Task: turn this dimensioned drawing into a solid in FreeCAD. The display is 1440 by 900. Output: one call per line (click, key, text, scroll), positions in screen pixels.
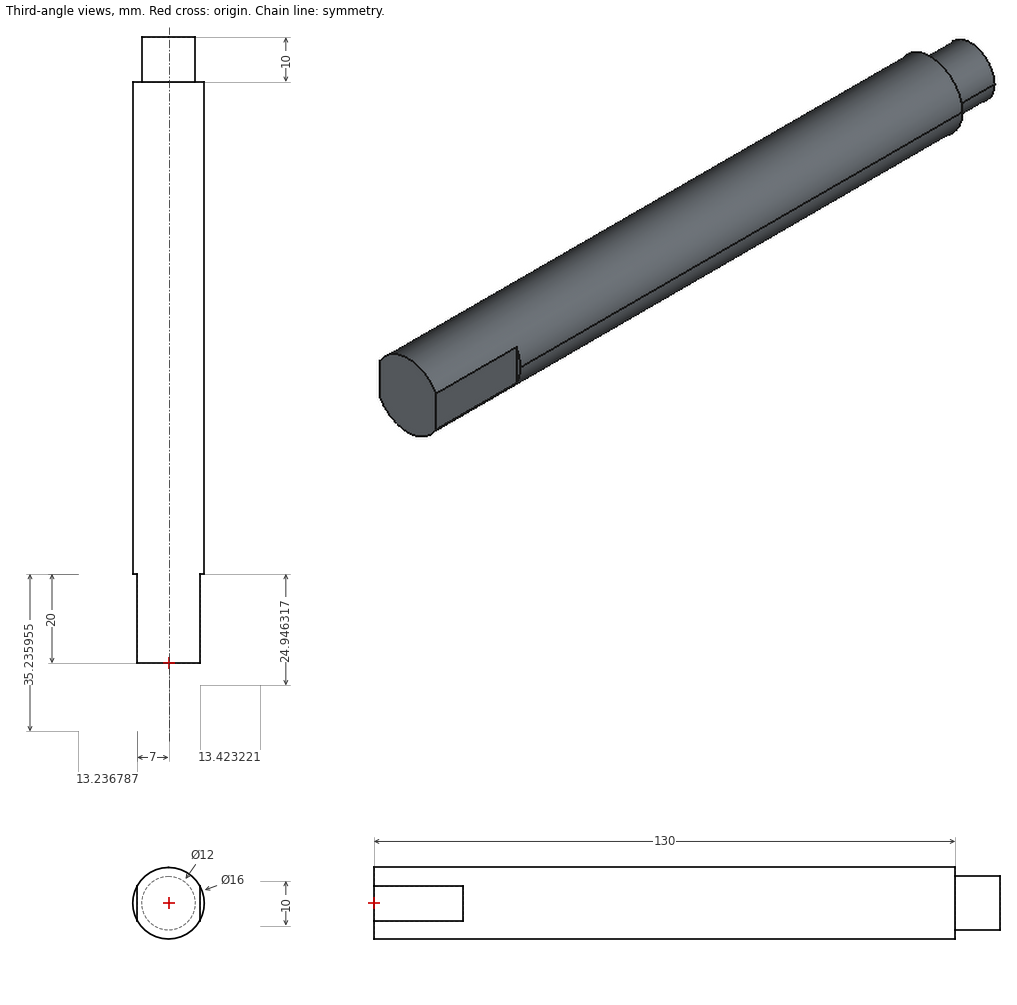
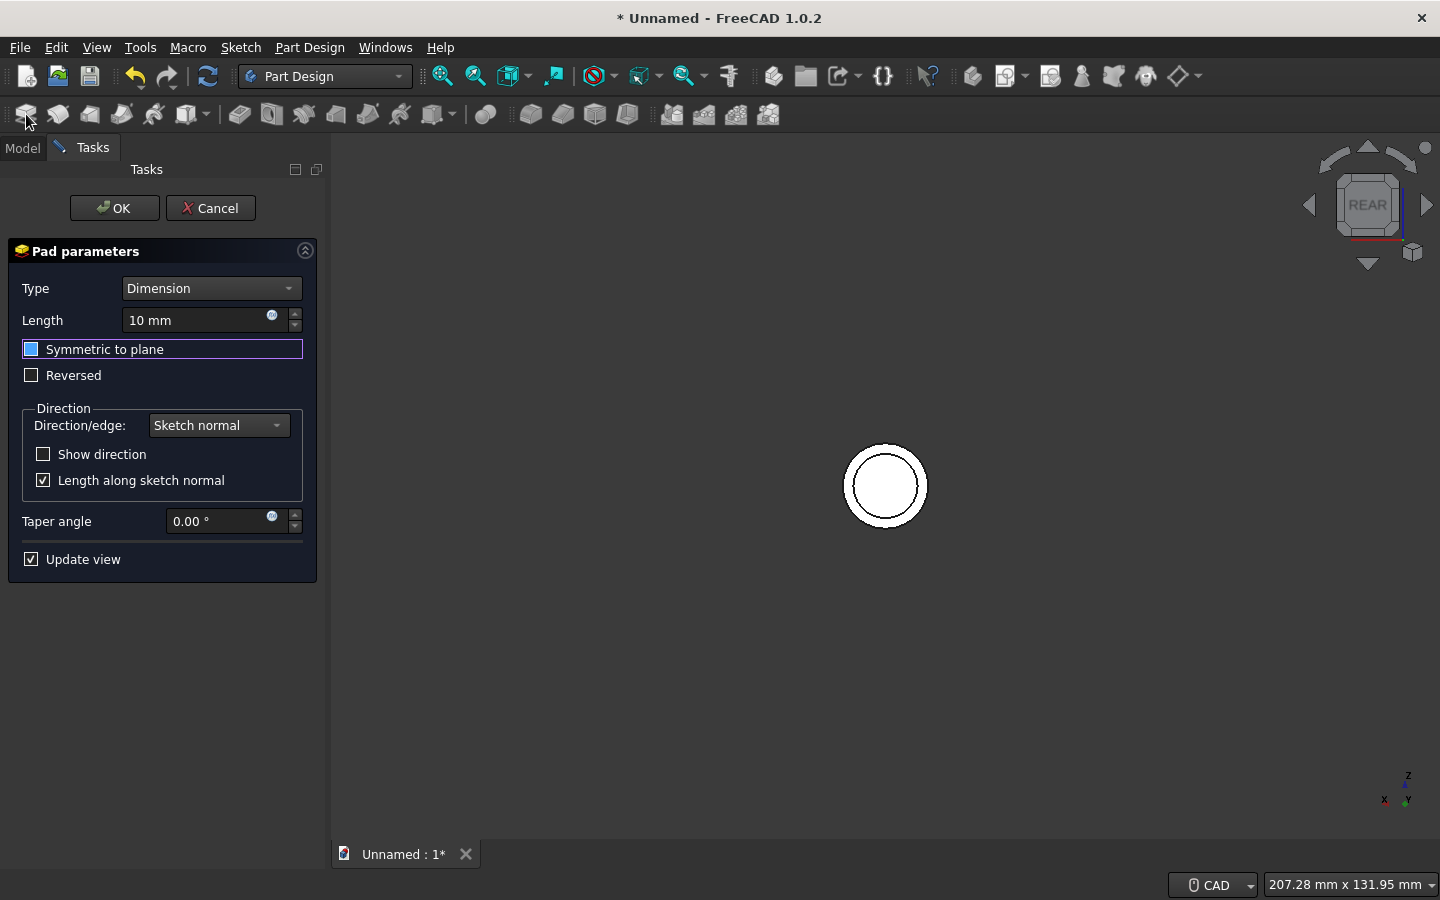
click(115, 208)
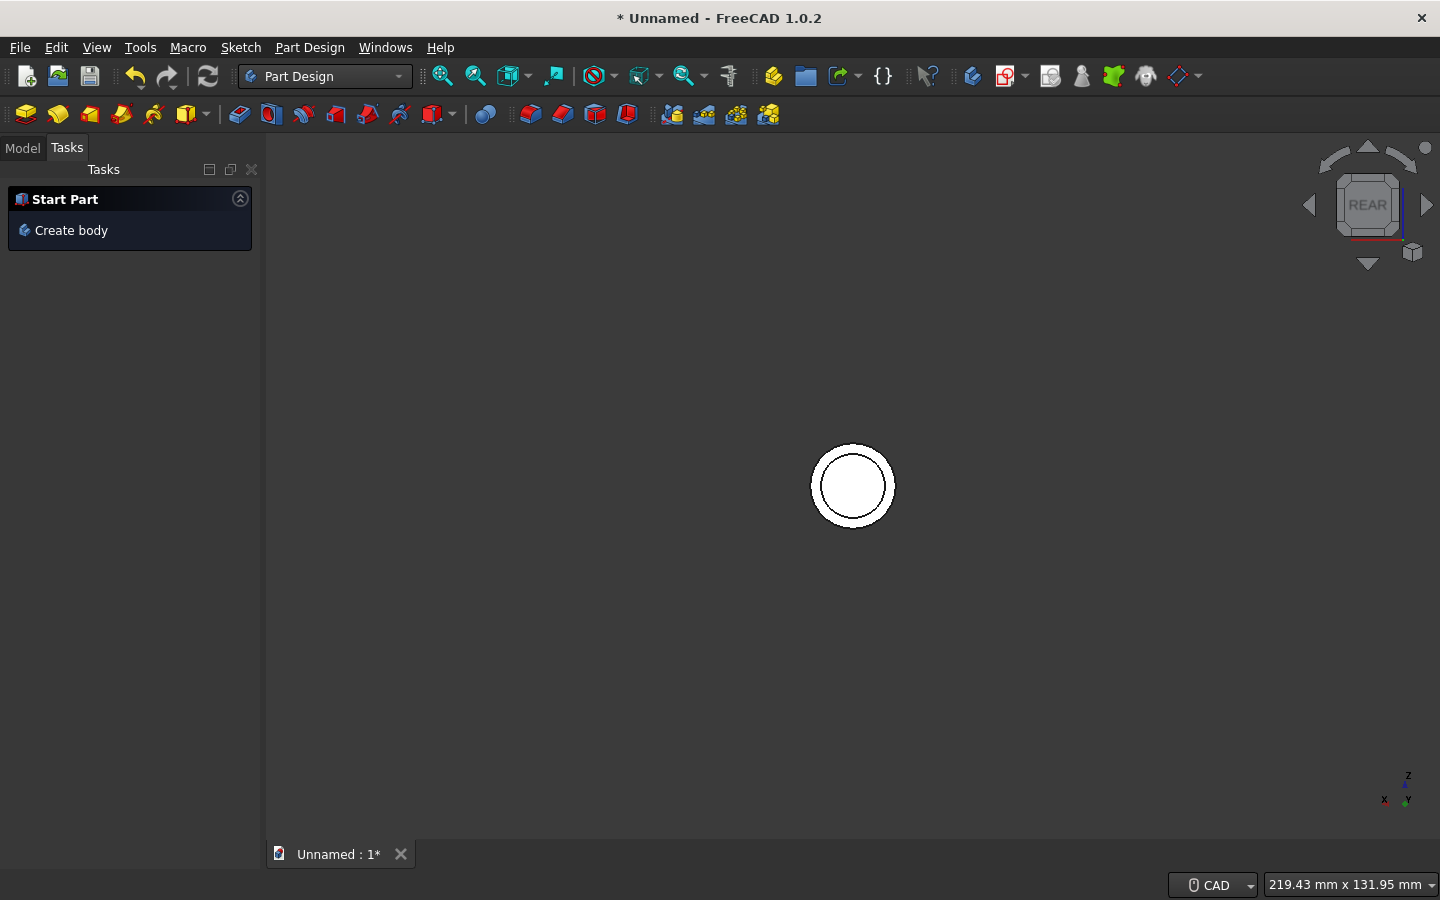
click(444, 76)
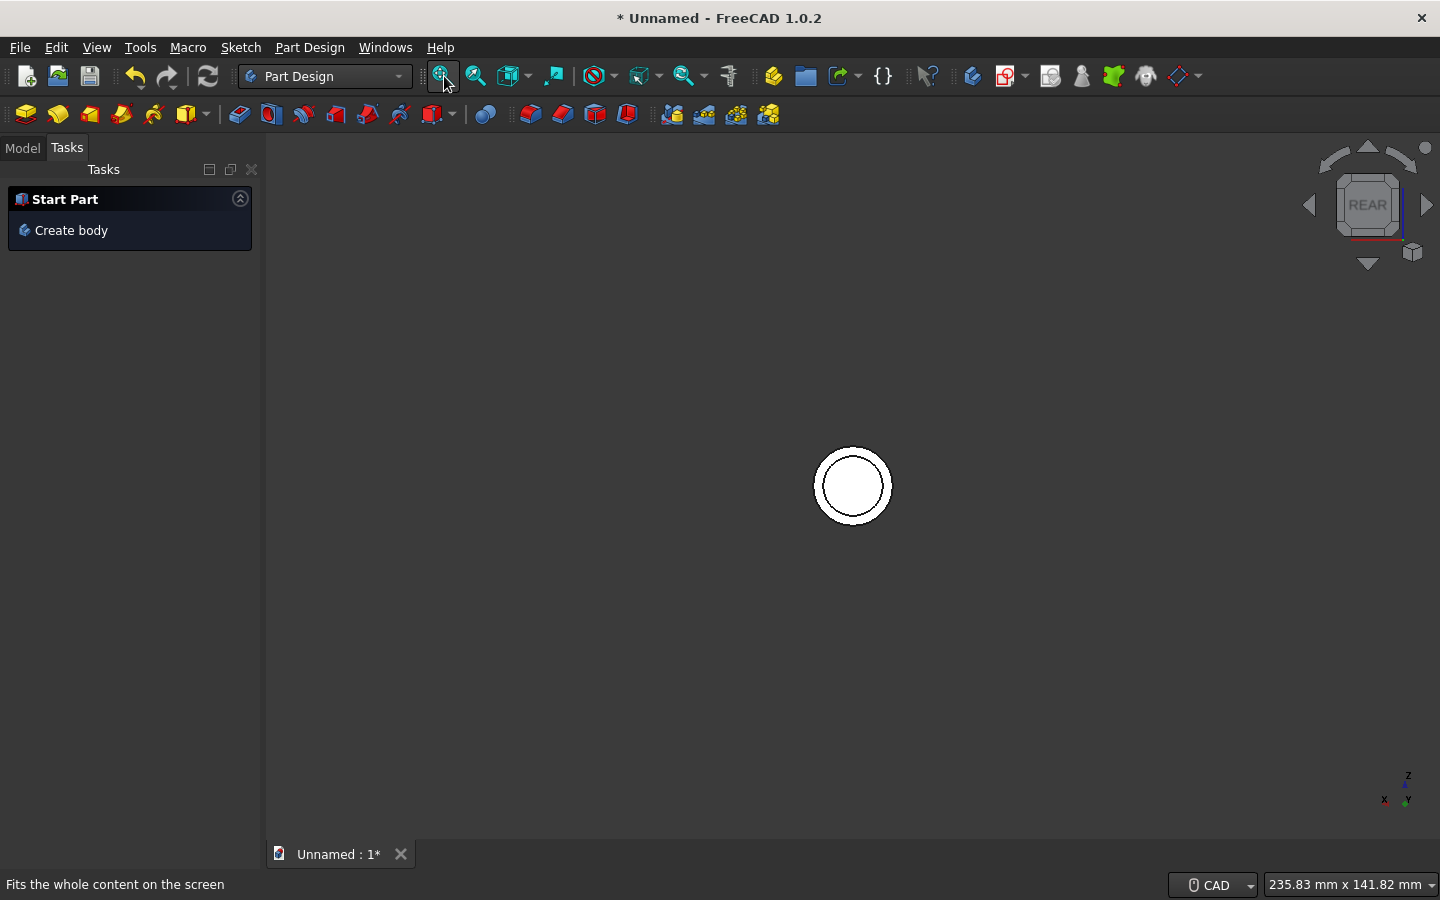
click(1006, 76)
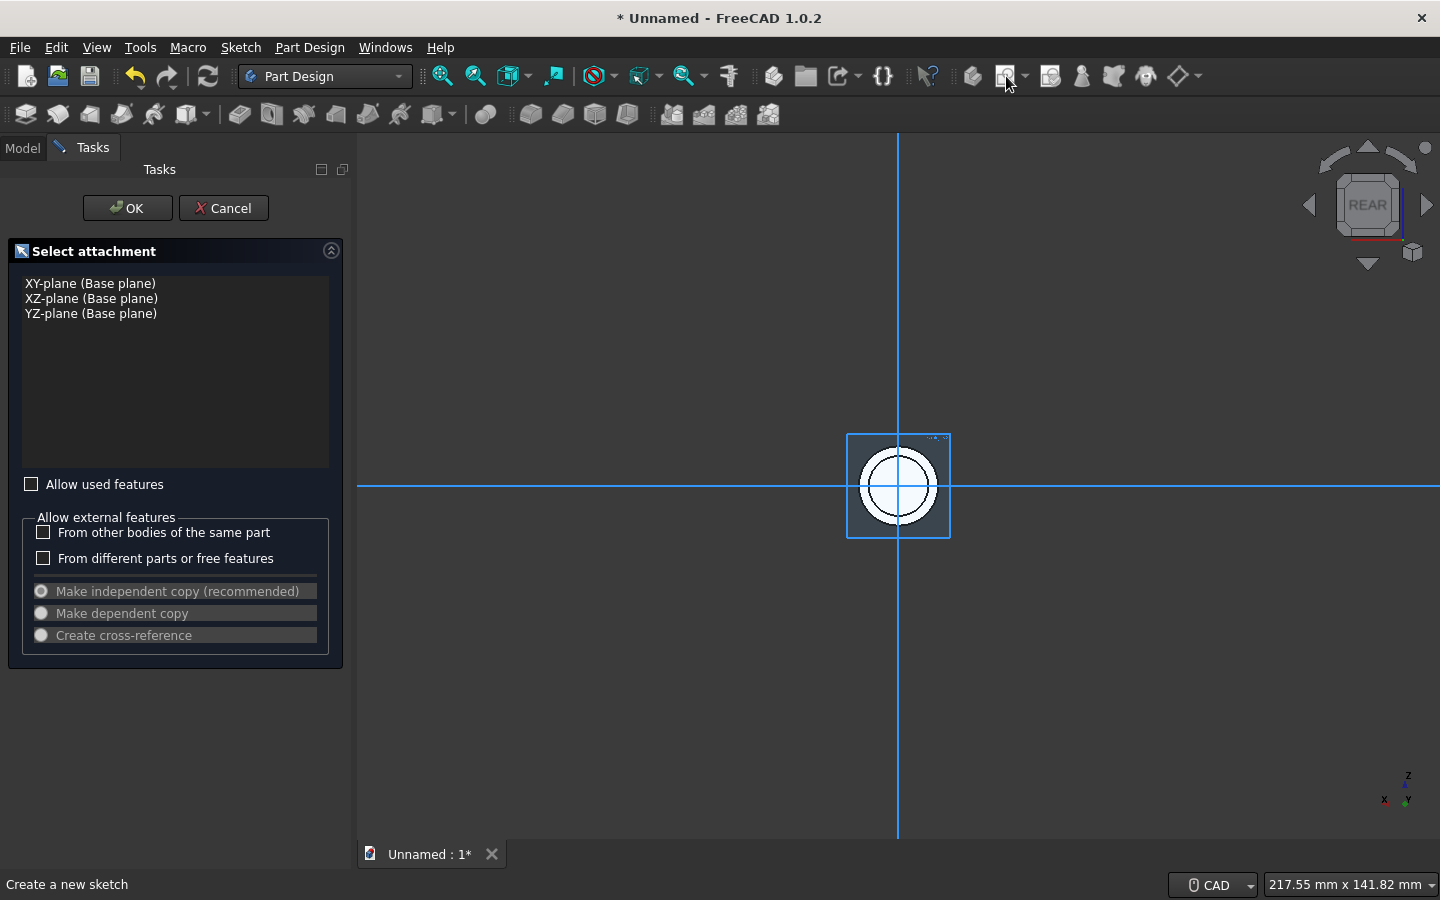
click(82, 284)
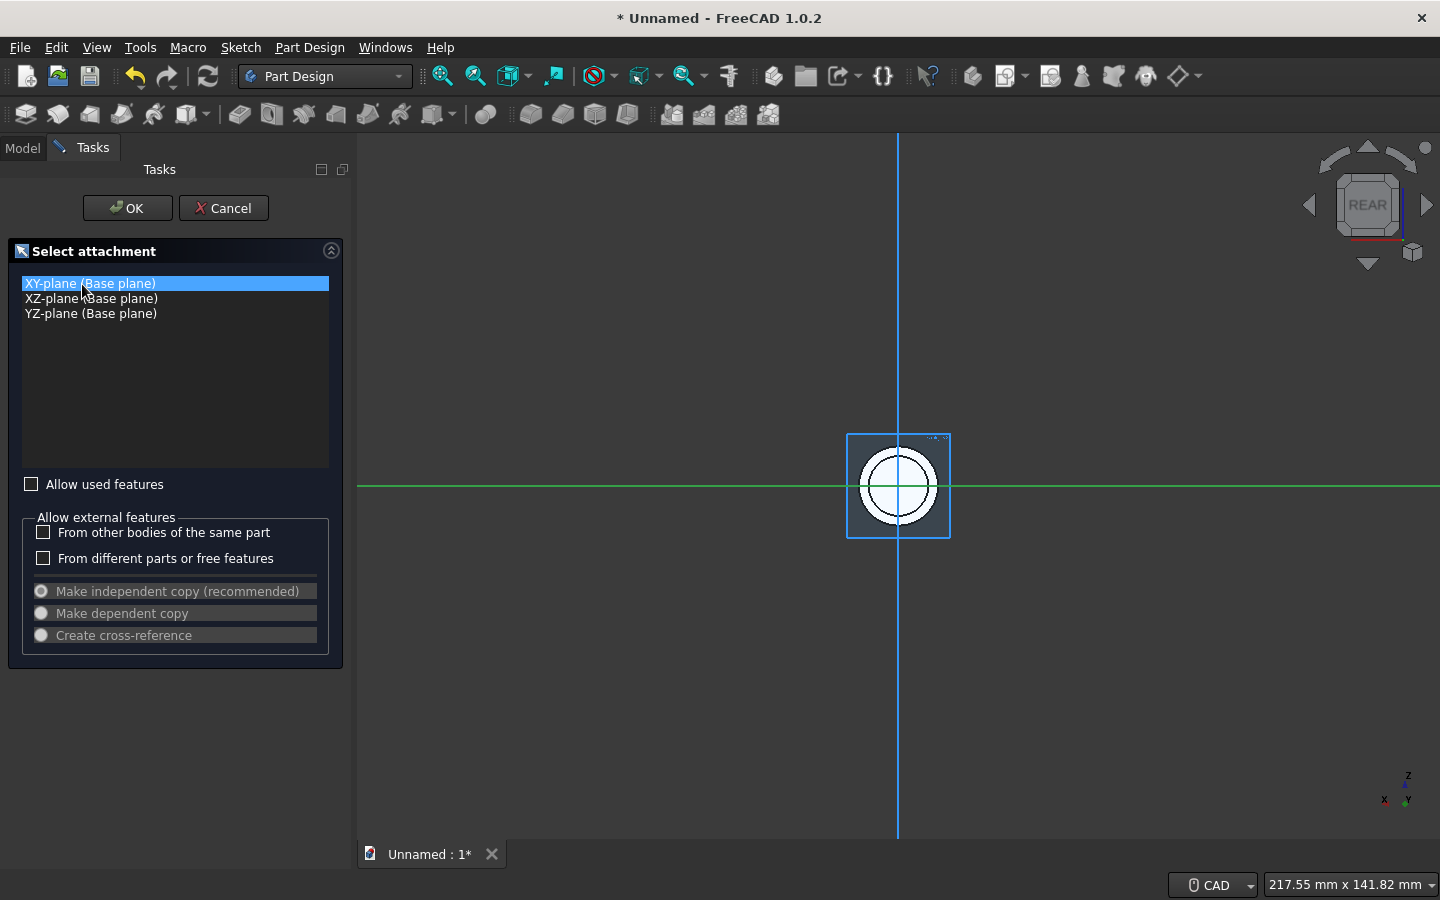
click(128, 208)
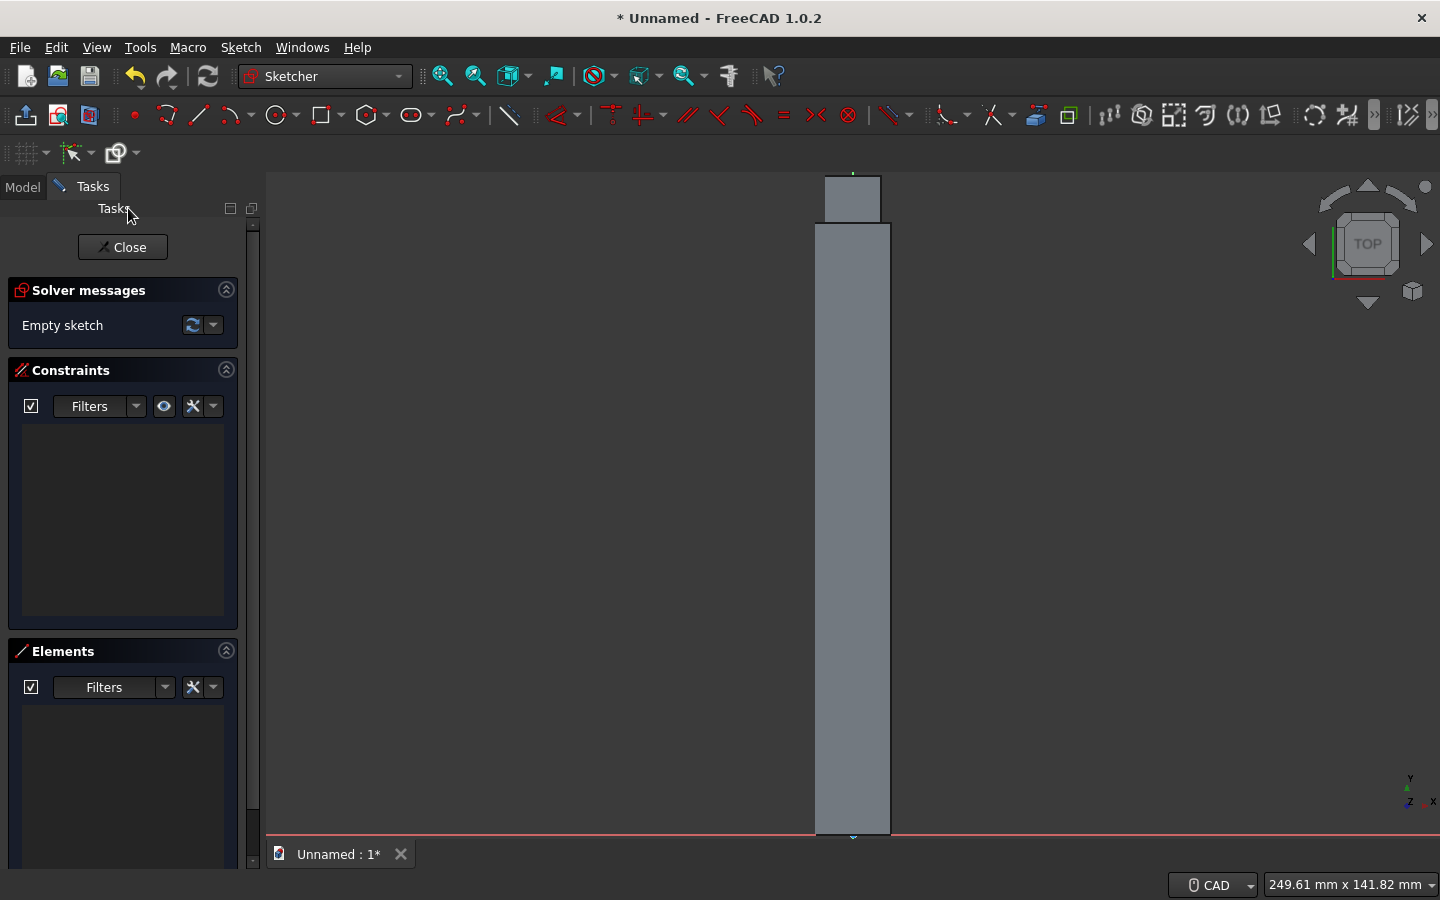
key(q)
key(s)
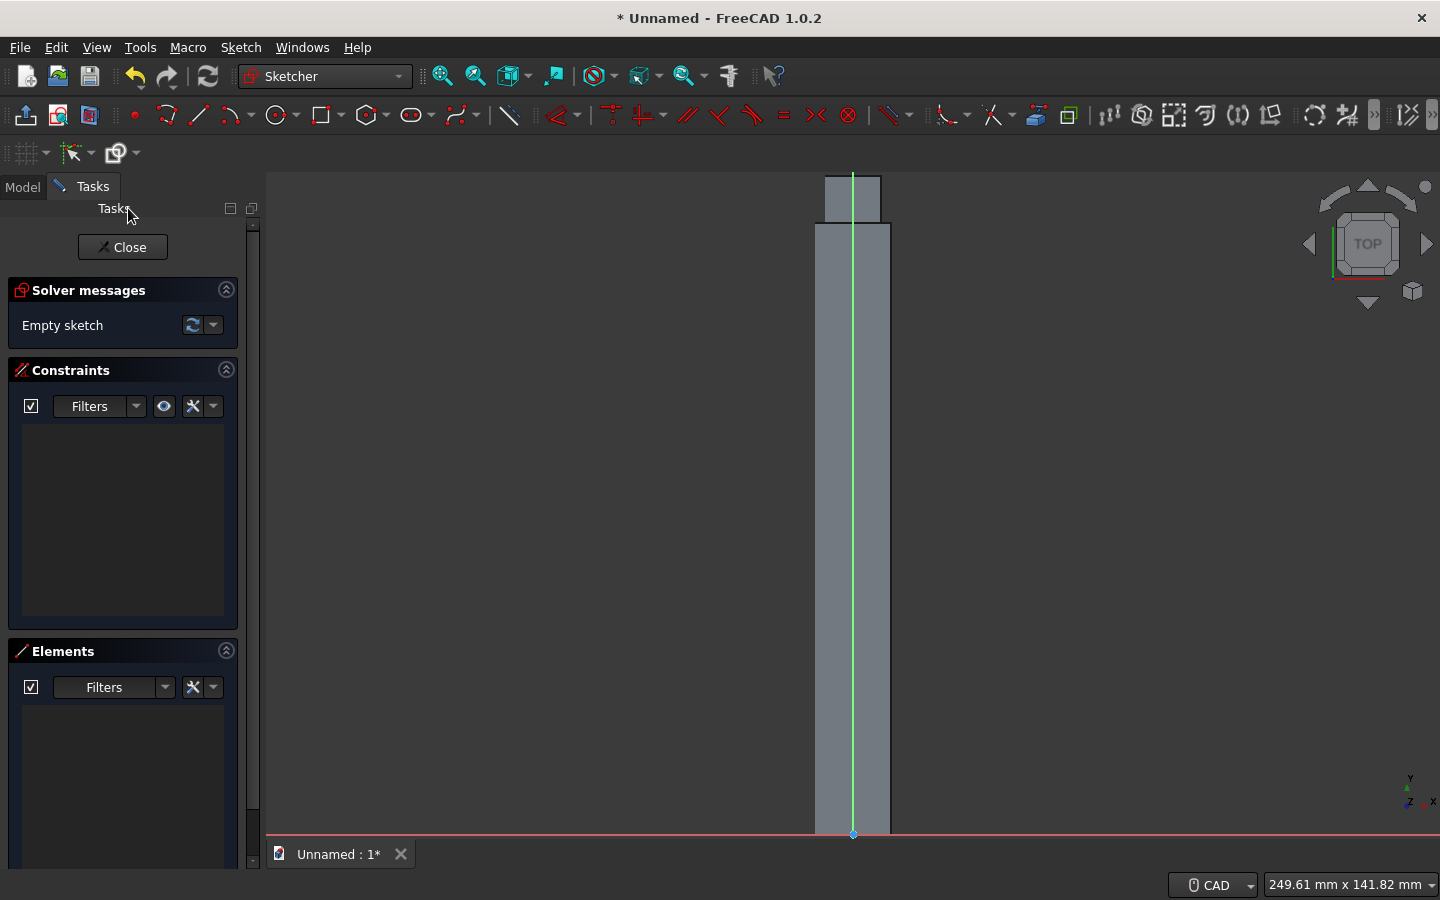
scroll(784, 506, down, 5)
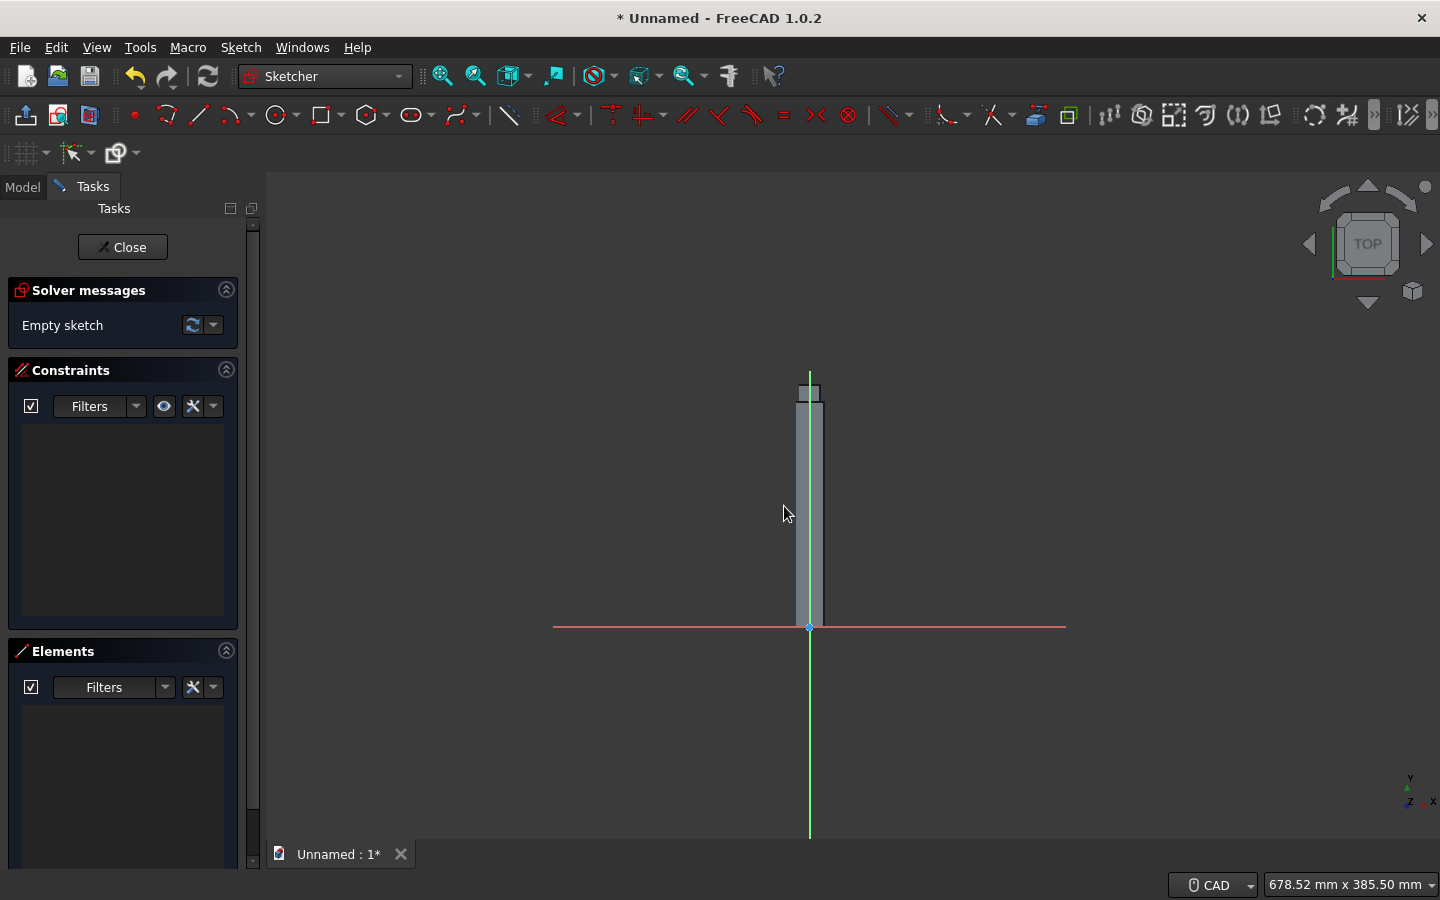
scroll(814, 642, up, 10)